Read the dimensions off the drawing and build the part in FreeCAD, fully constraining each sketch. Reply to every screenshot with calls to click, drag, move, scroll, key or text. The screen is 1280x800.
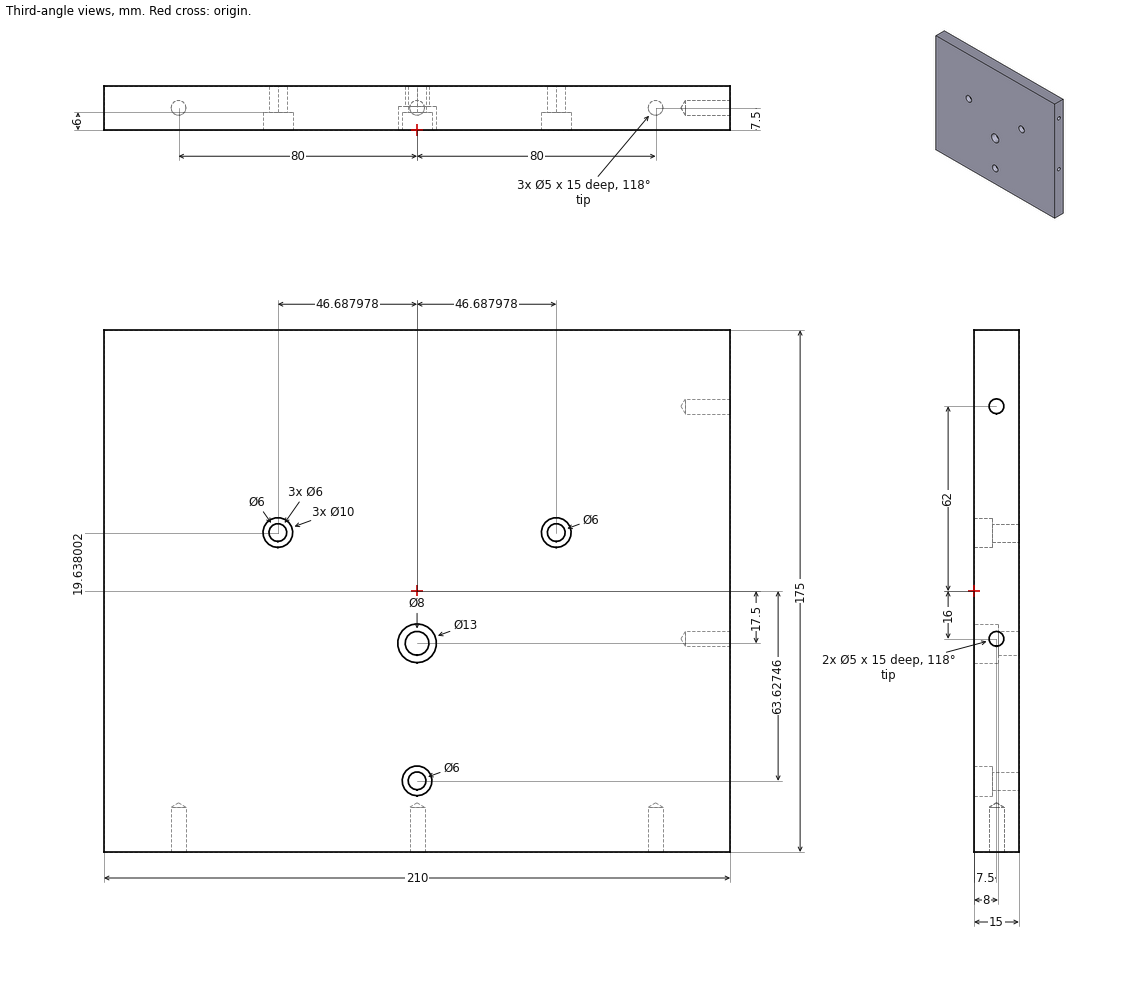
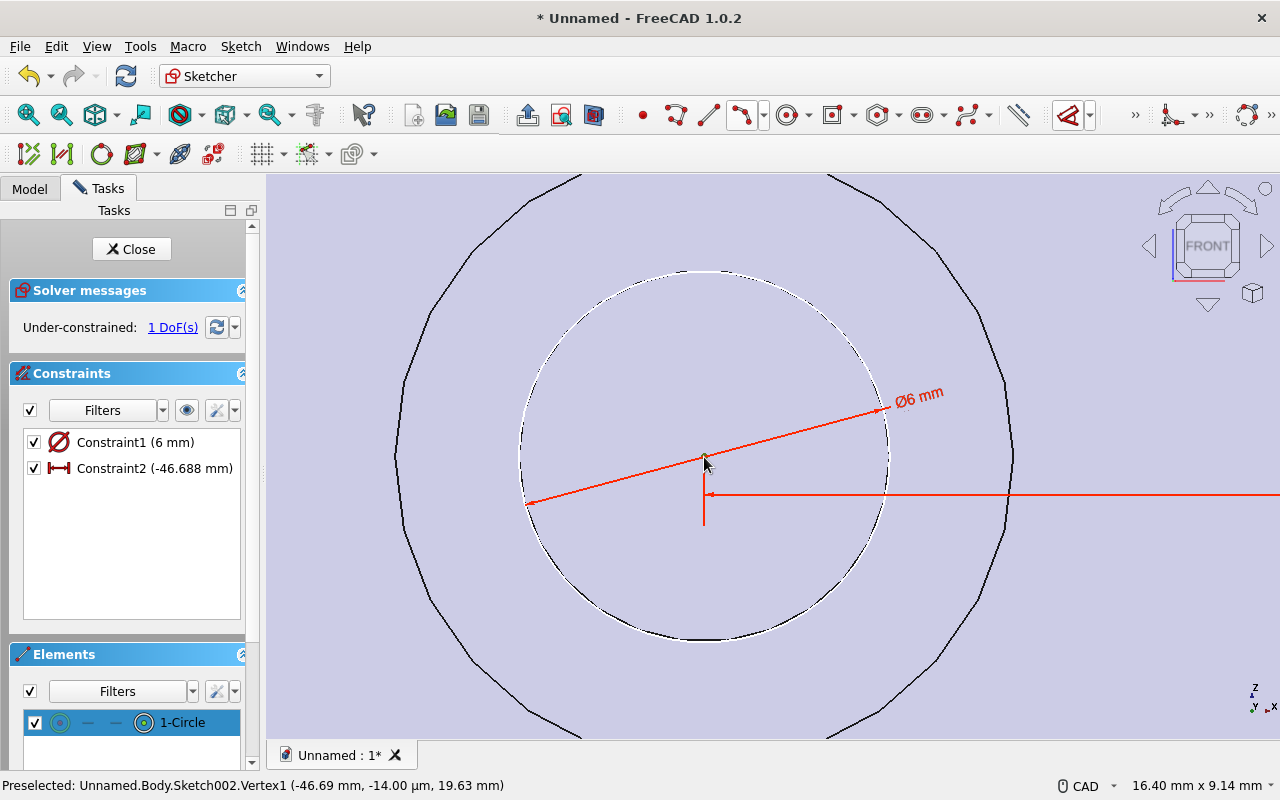
click(1090, 116)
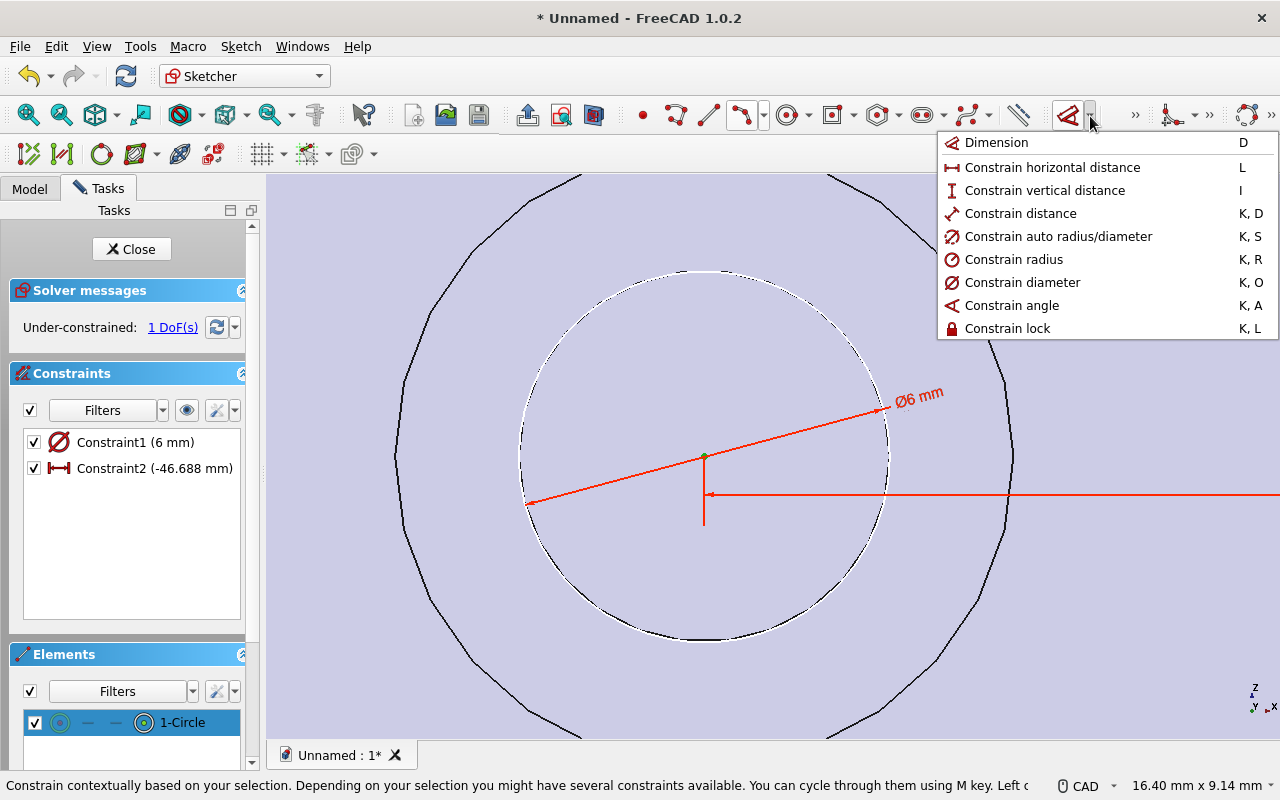
click(1108, 190)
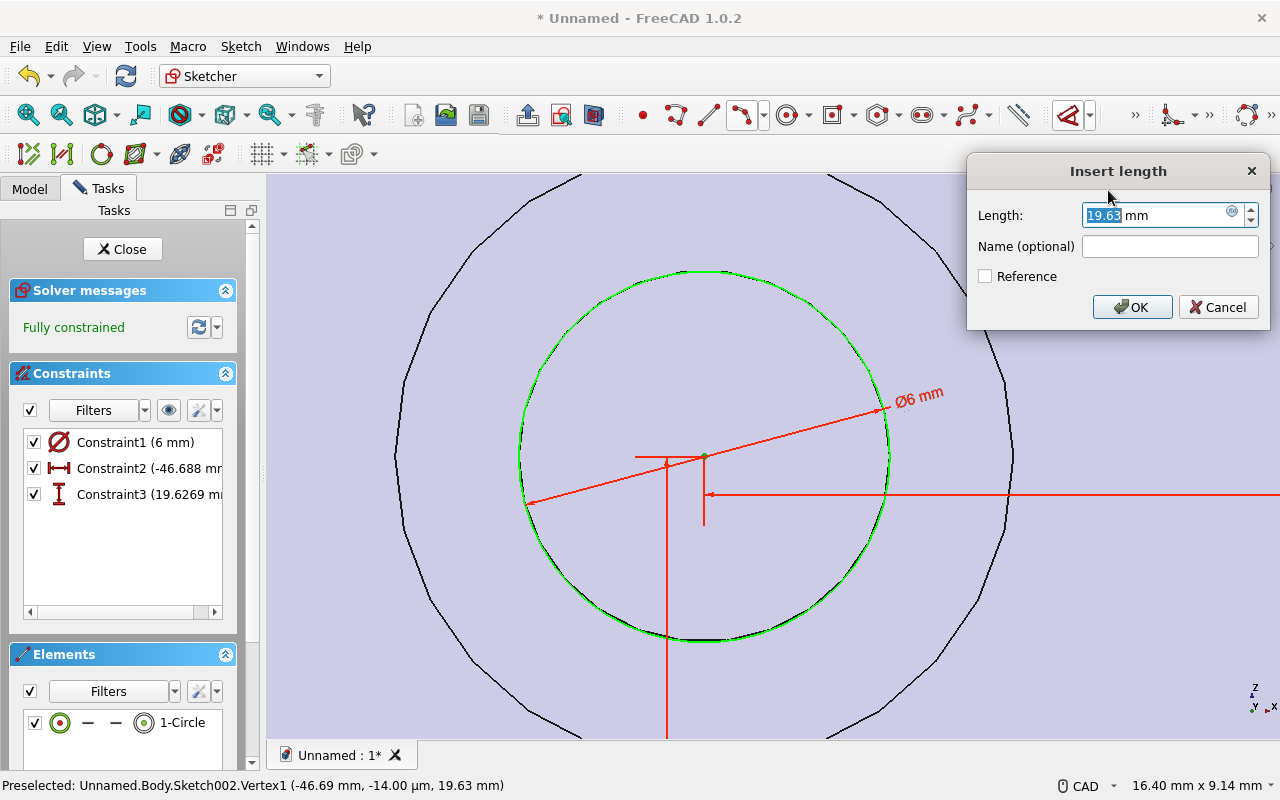
text(19.638002)
key(Return)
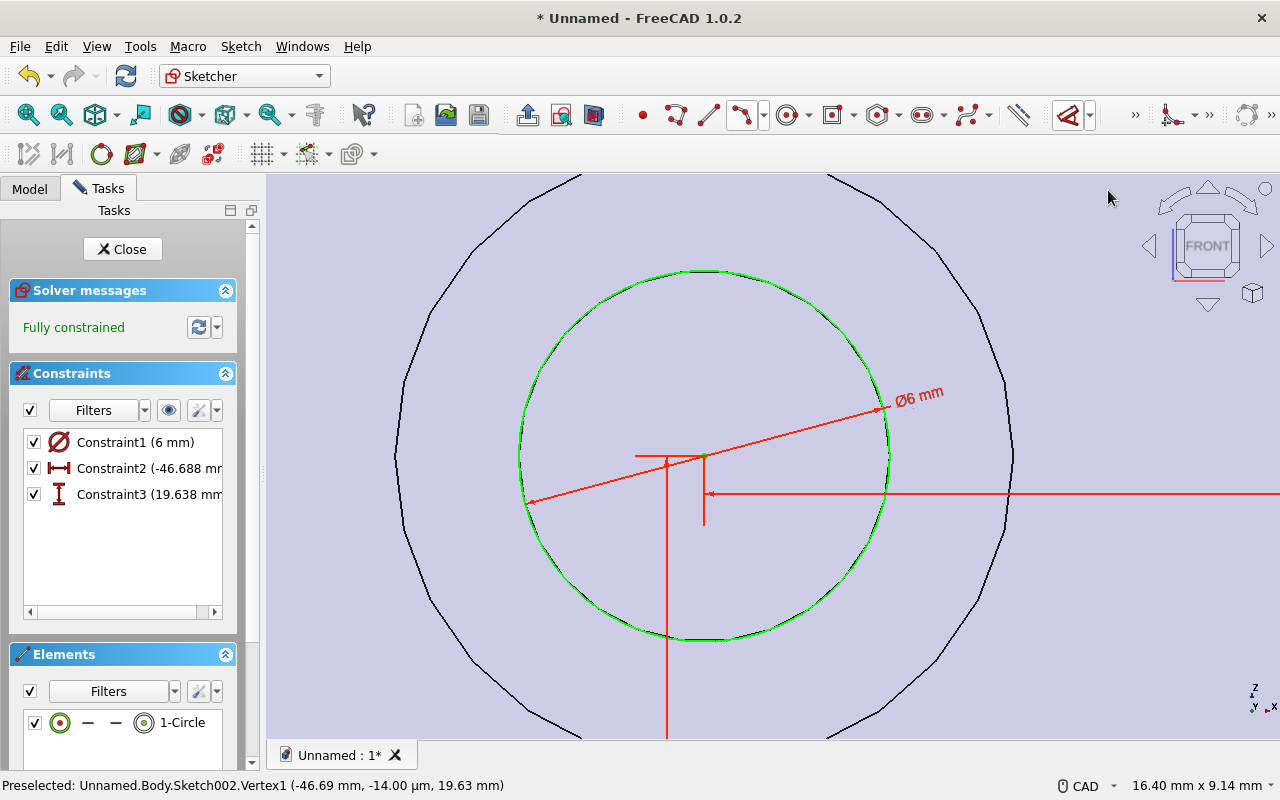
click(123, 249)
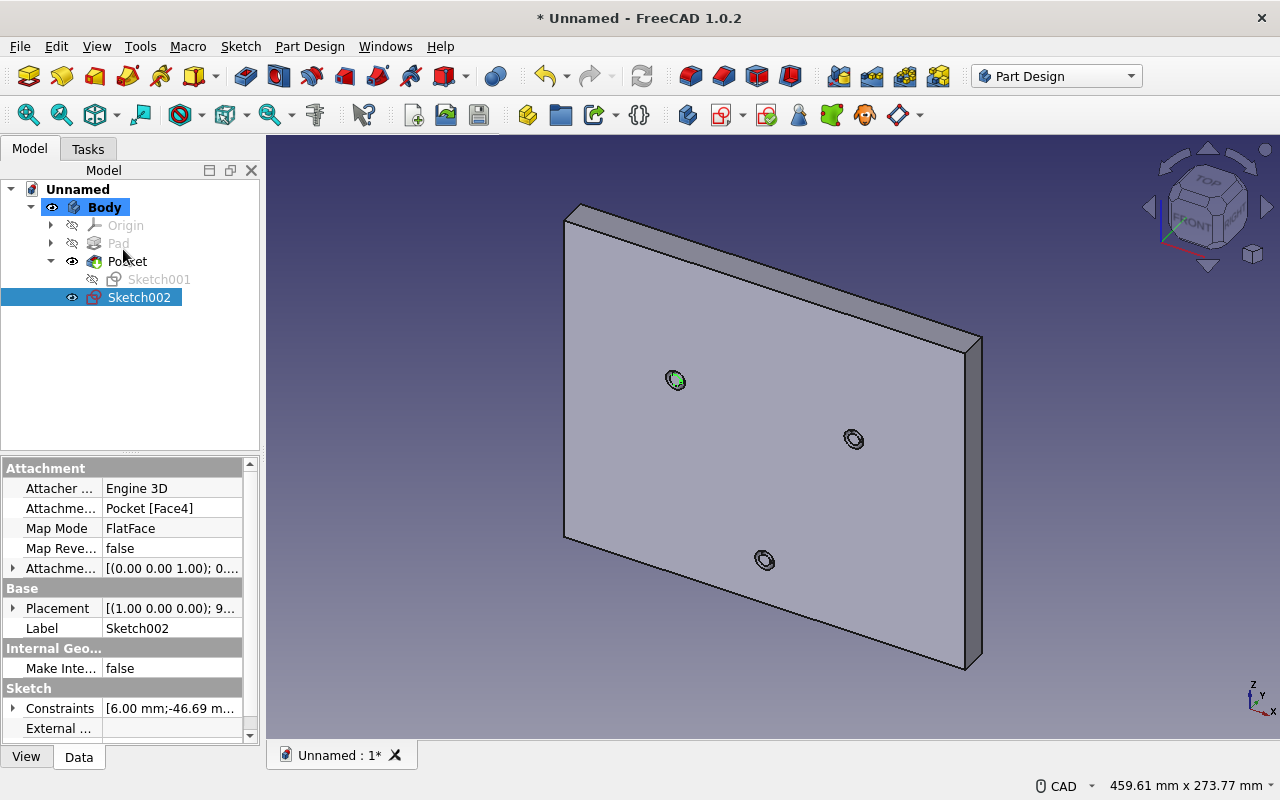
click(246, 76)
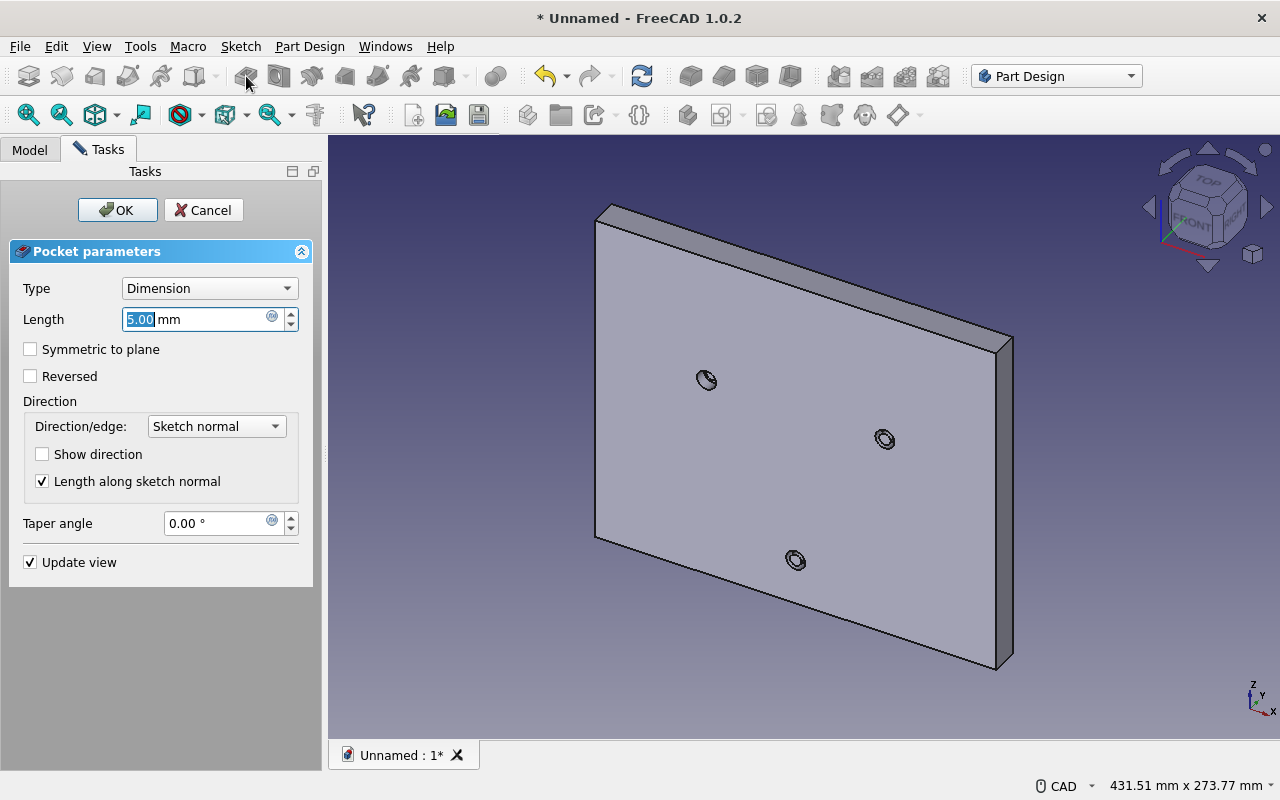
click(210, 288)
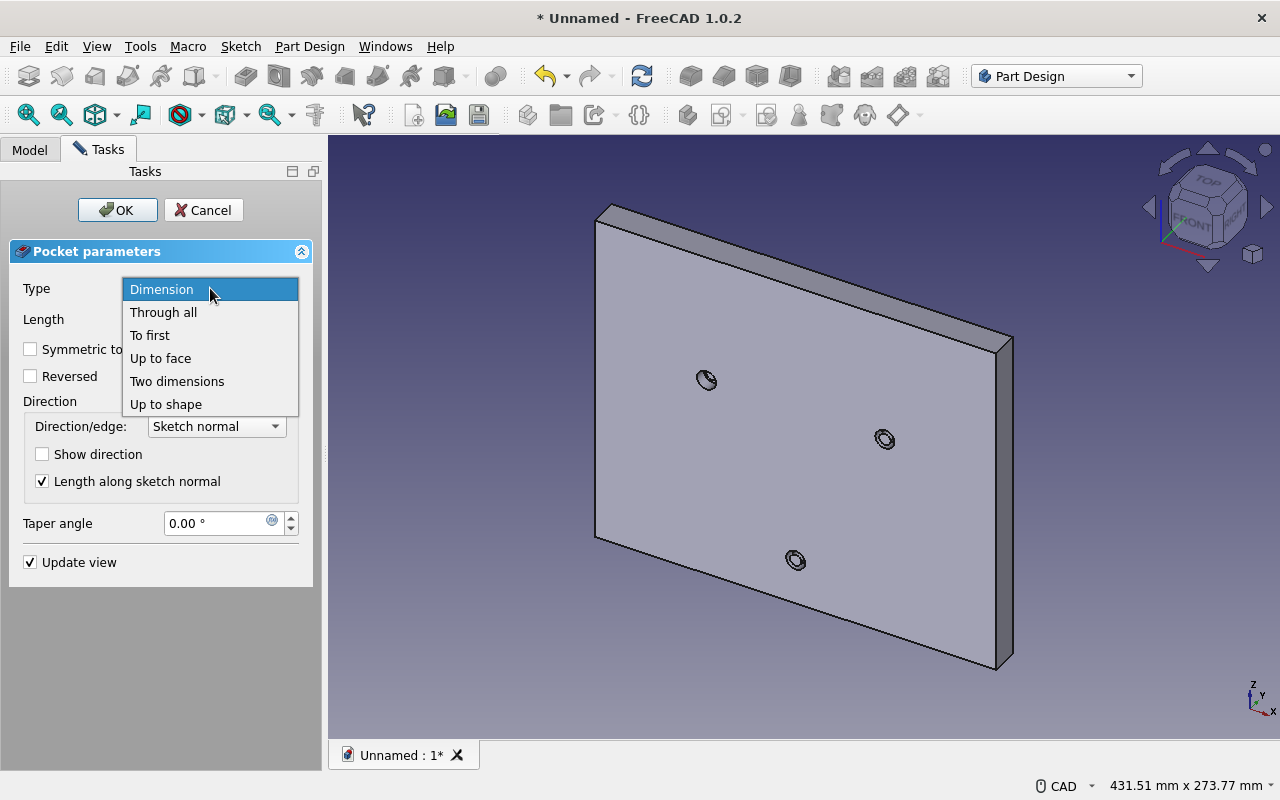
click(208, 336)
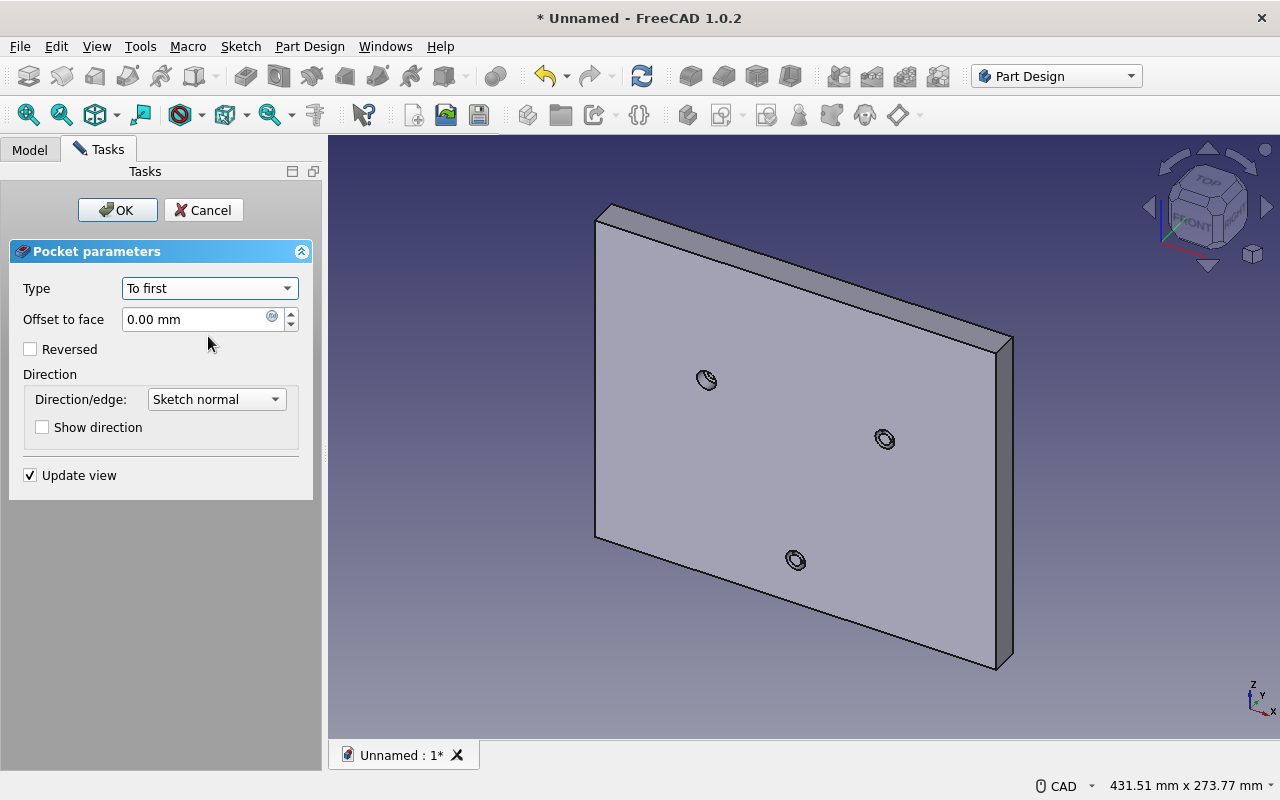
click(118, 210)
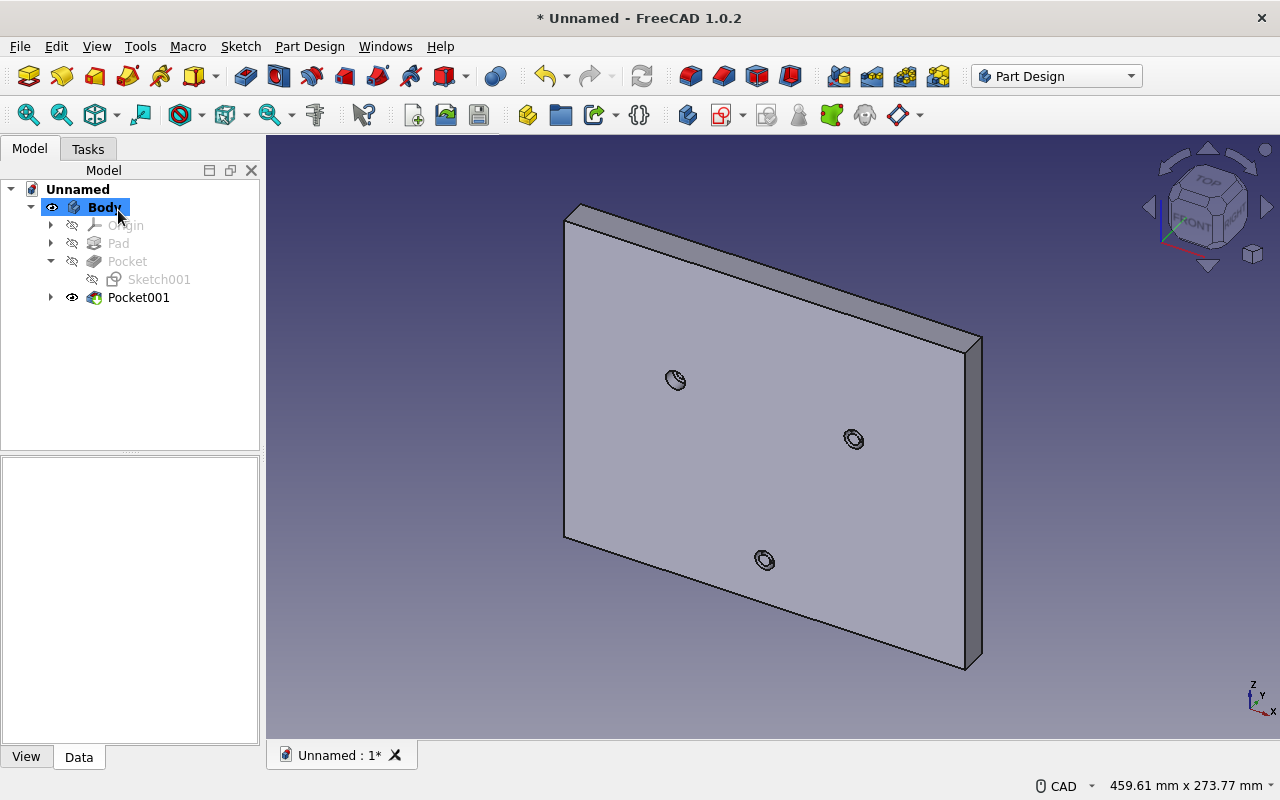
click(720, 116)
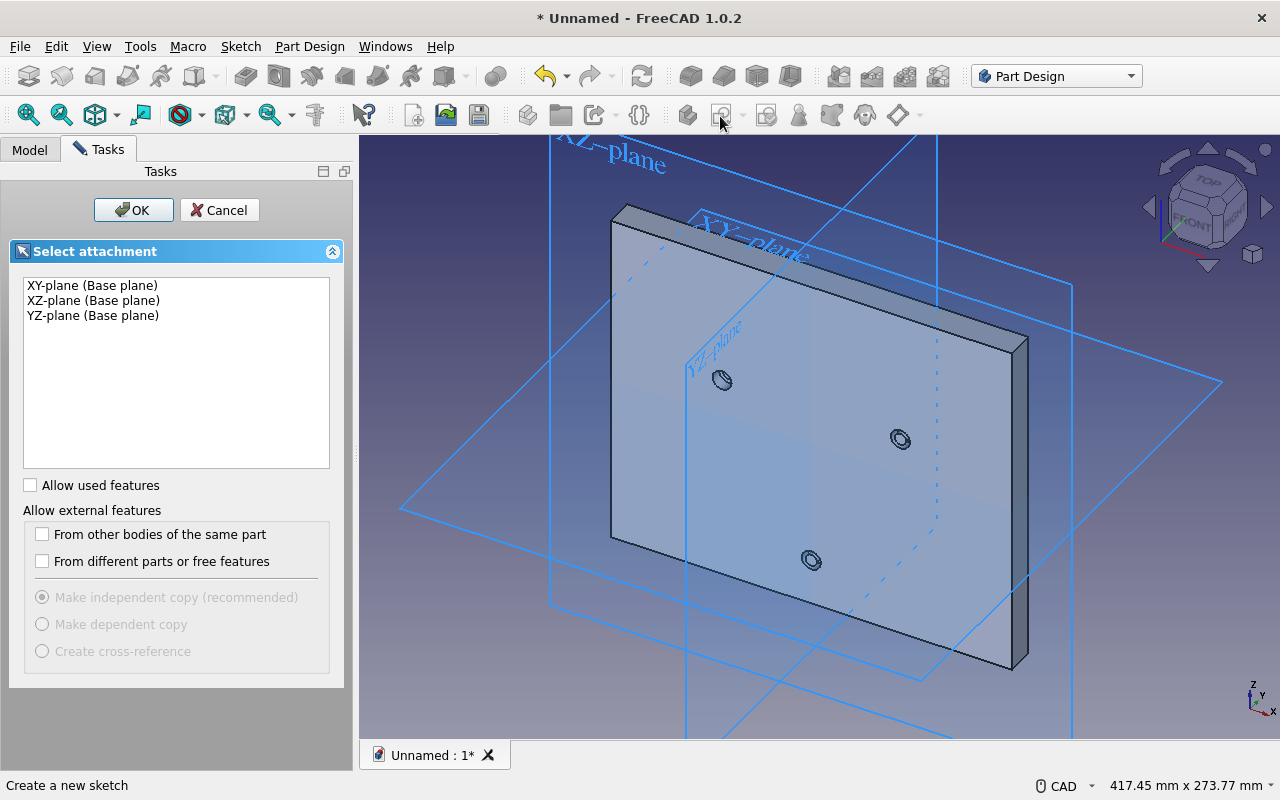
click(84, 300)